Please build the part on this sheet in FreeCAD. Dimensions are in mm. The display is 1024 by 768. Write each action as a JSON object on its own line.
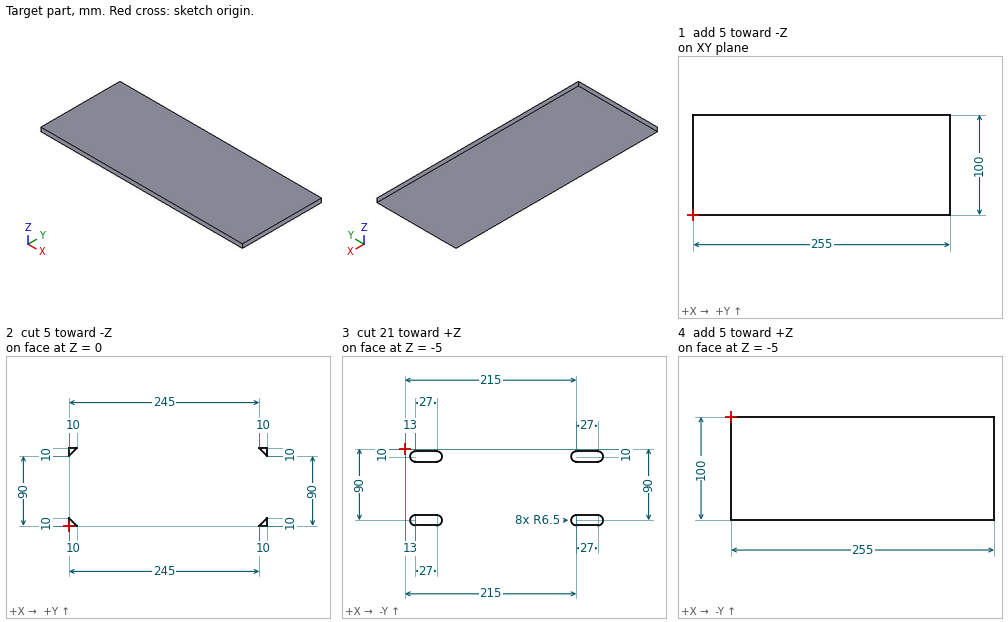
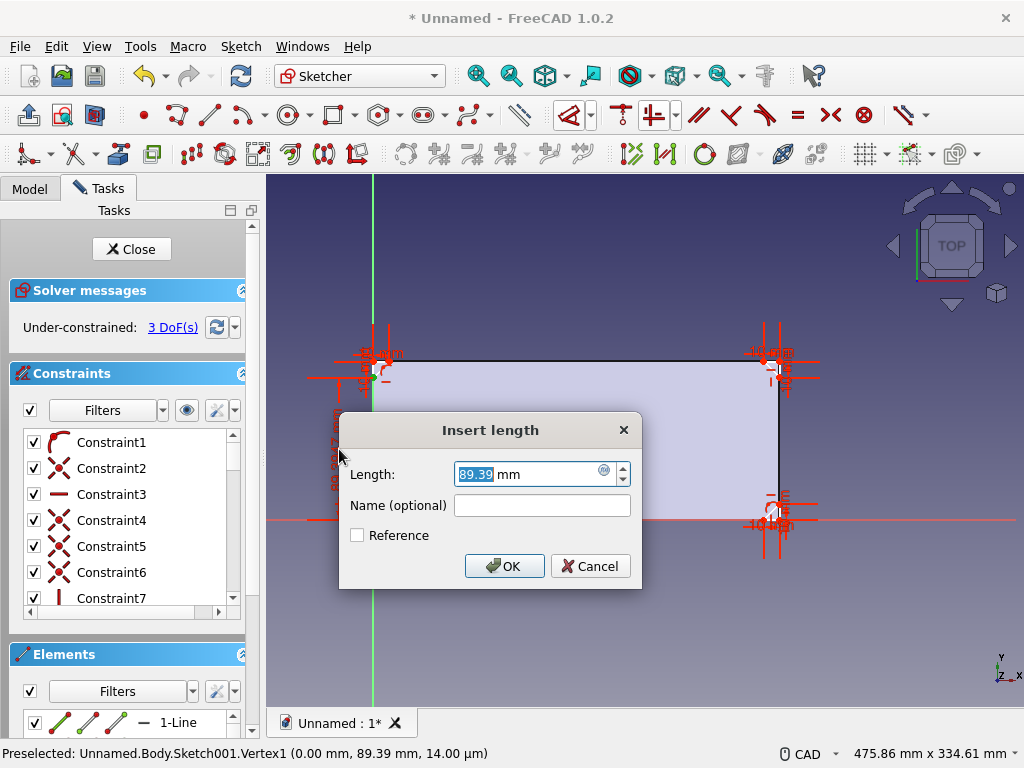
{"action": "type", "text": "90"}
{"action": "key", "text": "Return"}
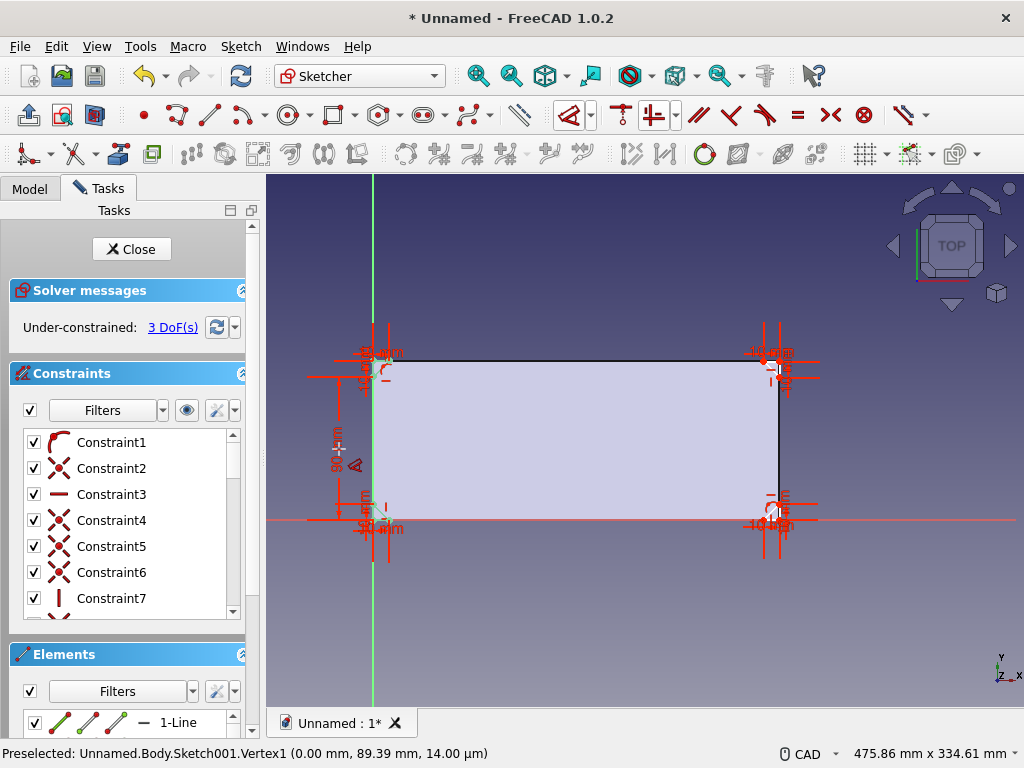
{"action": "left_click", "coordinate": [780, 378]}
{"action": "left_click", "coordinate": [814, 449]}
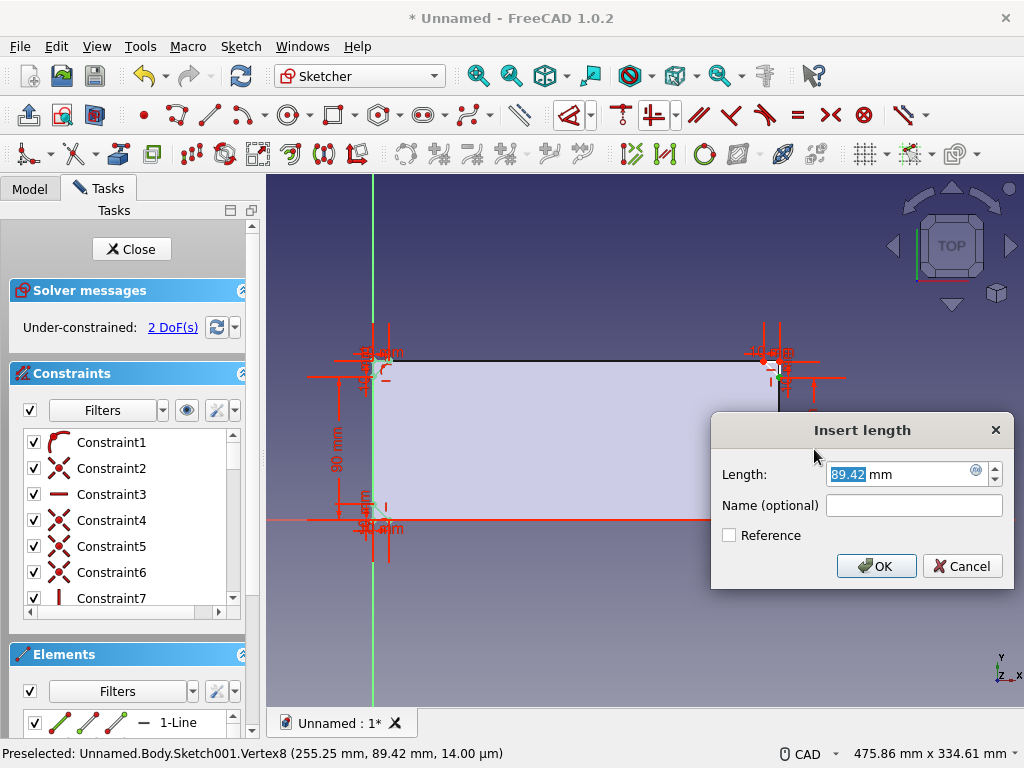
{"action": "type", "text": "90"}
{"action": "key", "text": "Return"}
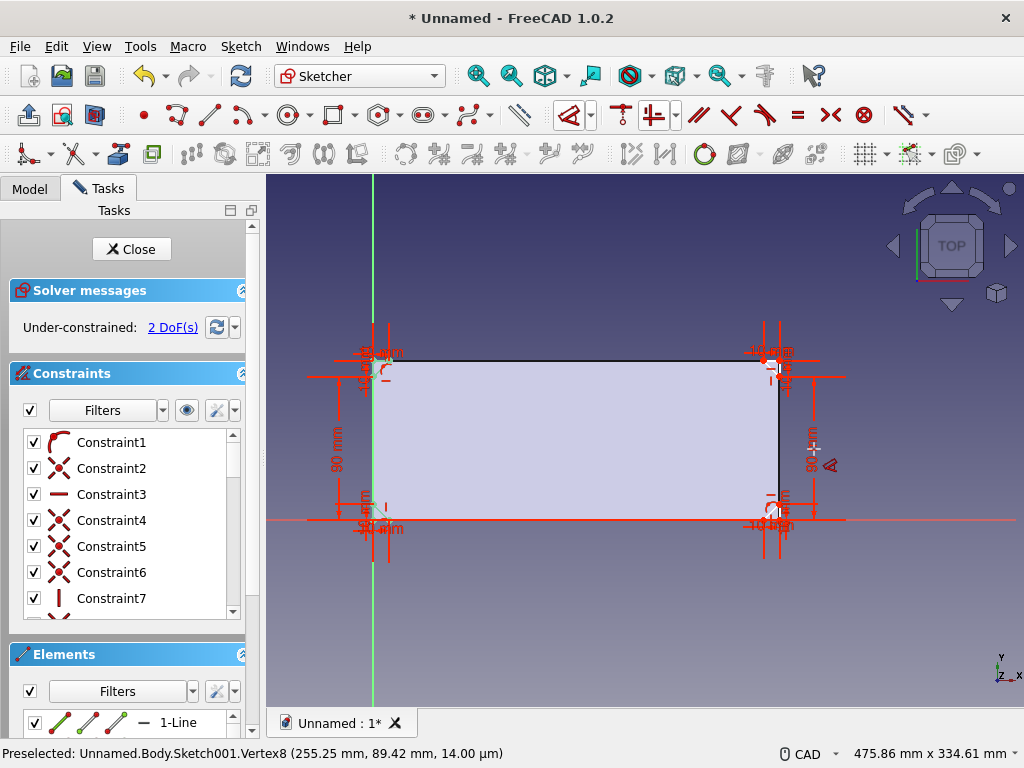
{"action": "left_click", "coordinate": [764, 361]}
{"action": "left_click", "coordinate": [569, 554]}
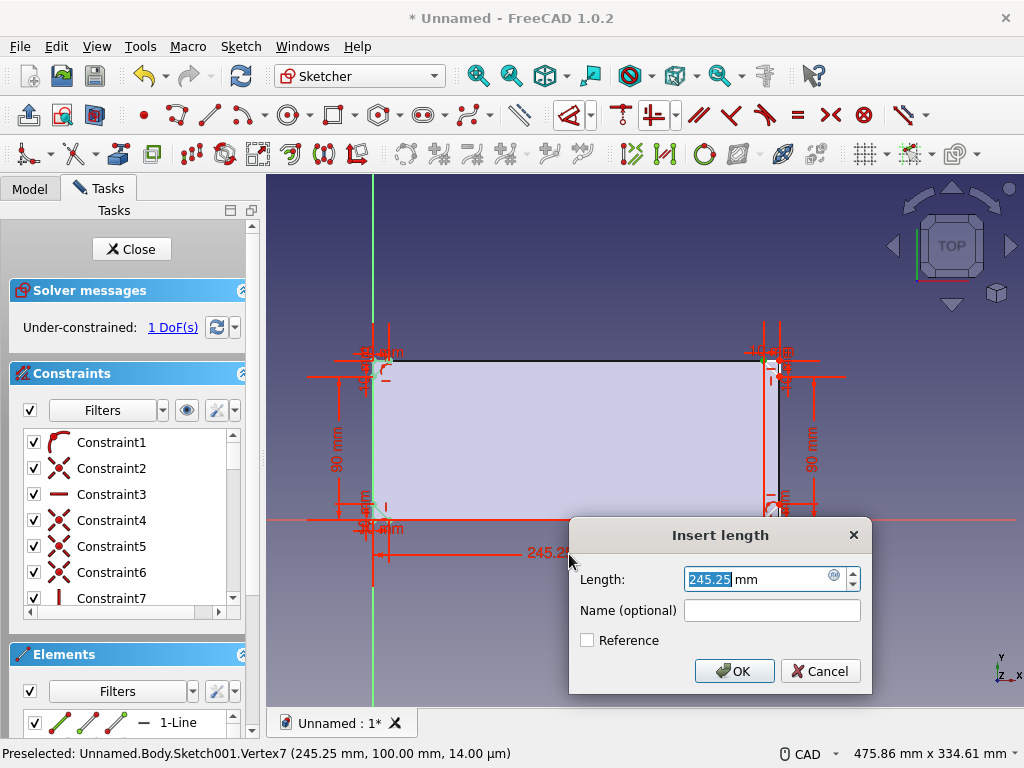
{"action": "type", "text": "245"}
{"action": "key", "text": "Return"}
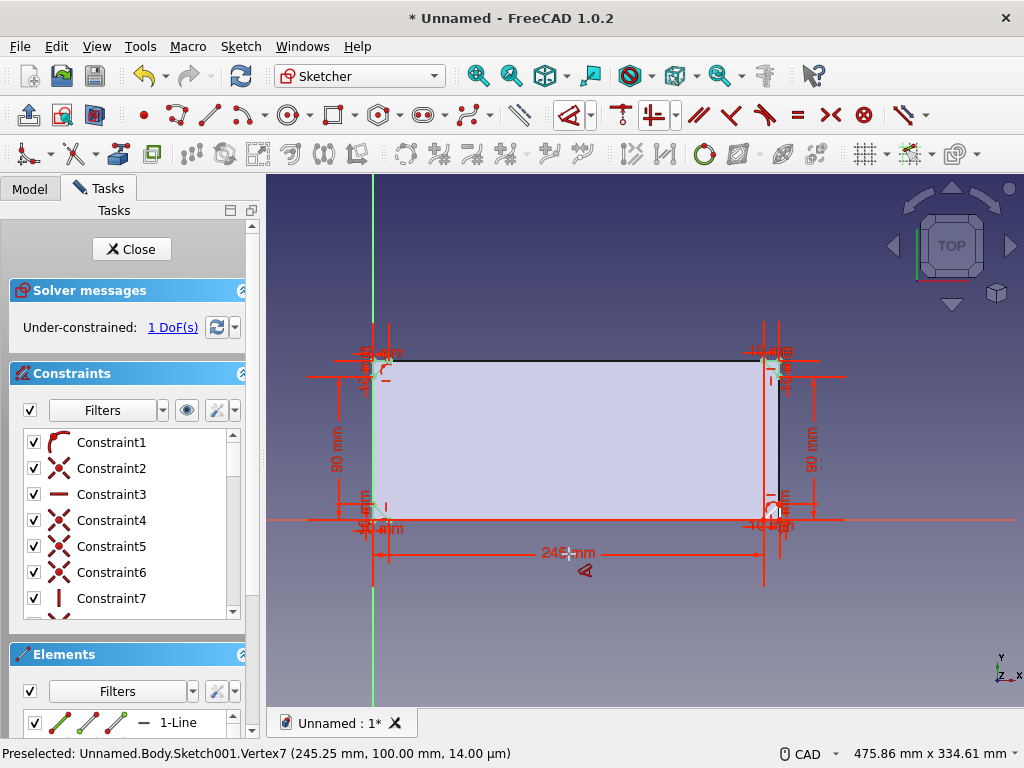
{"action": "left_click", "coordinate": [764, 520]}
{"action": "left_click", "coordinate": [479, 554]}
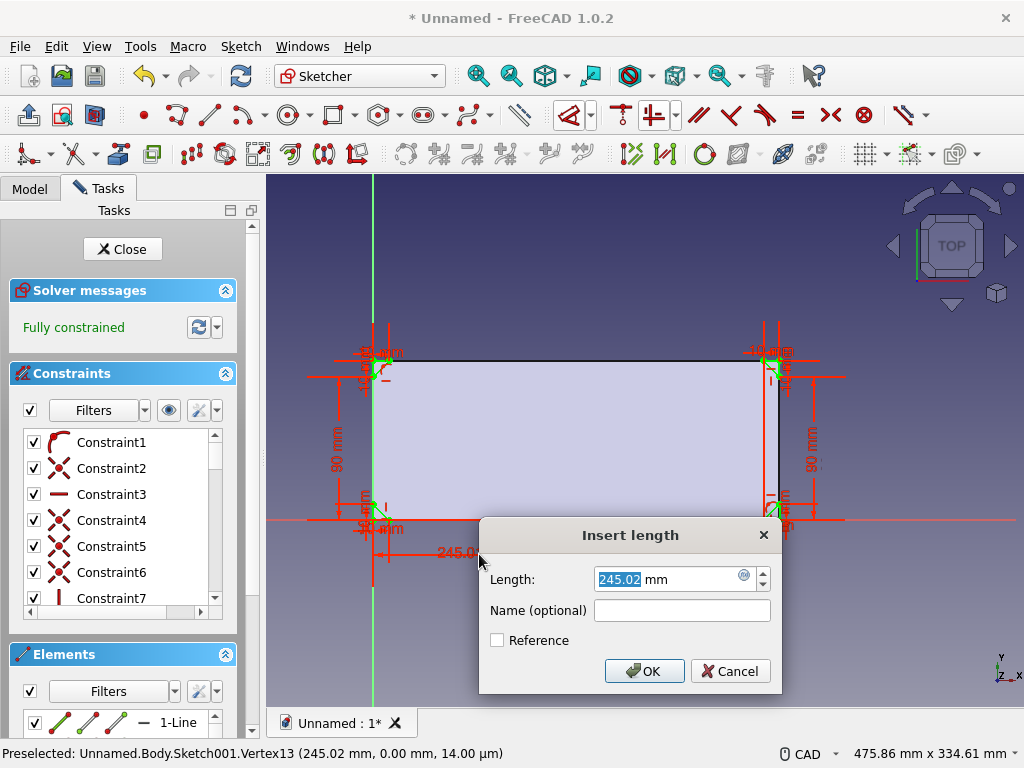
{"action": "type", "text": "245"}
{"action": "key", "text": "Return"}
{"action": "key", "text": "Escape"}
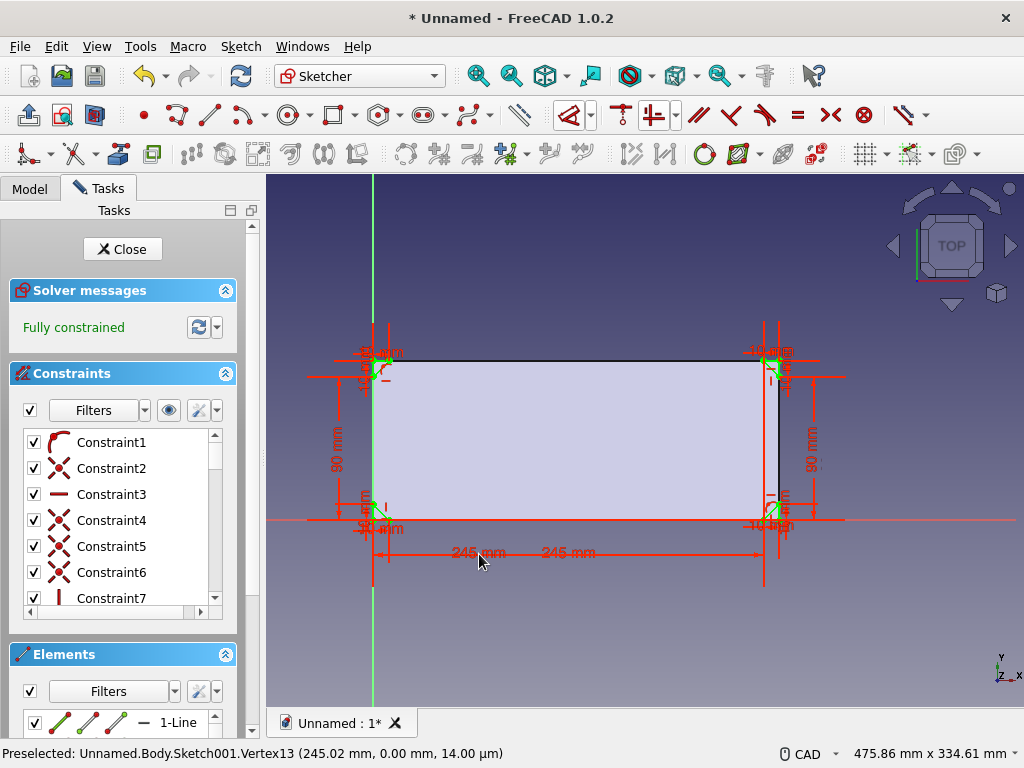
{"action": "left_click", "coordinate": [123, 249]}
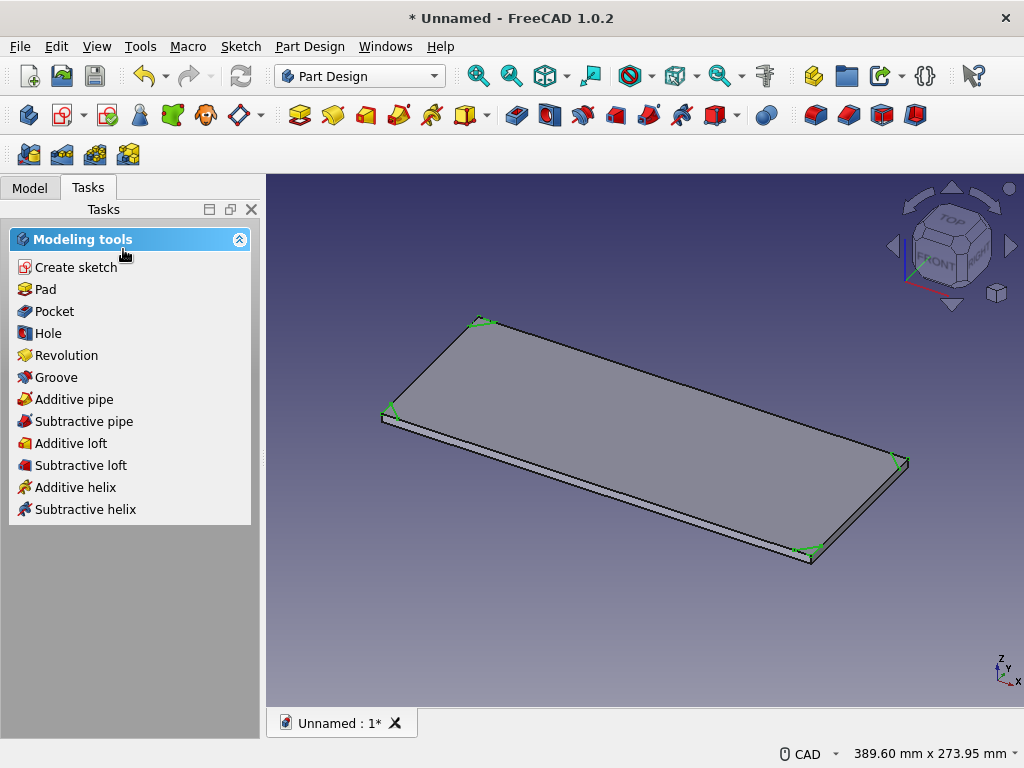
{"action": "left_click", "coordinate": [517, 116]}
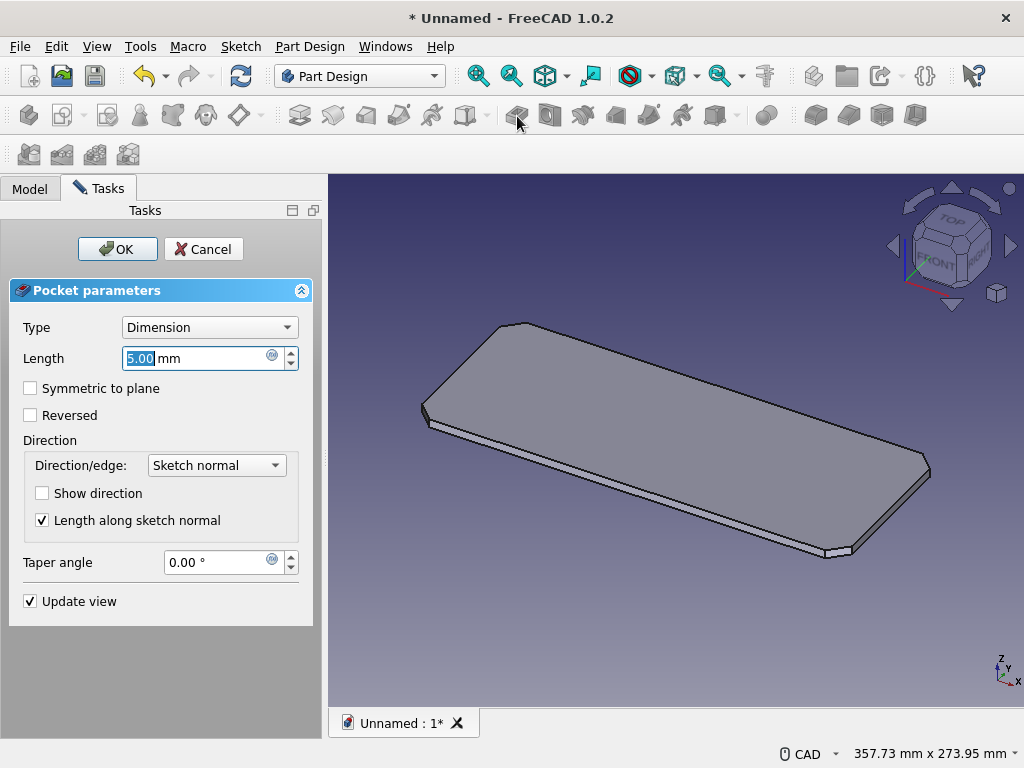
{"action": "type", "text": "5"}
{"action": "key", "text": "Tab"}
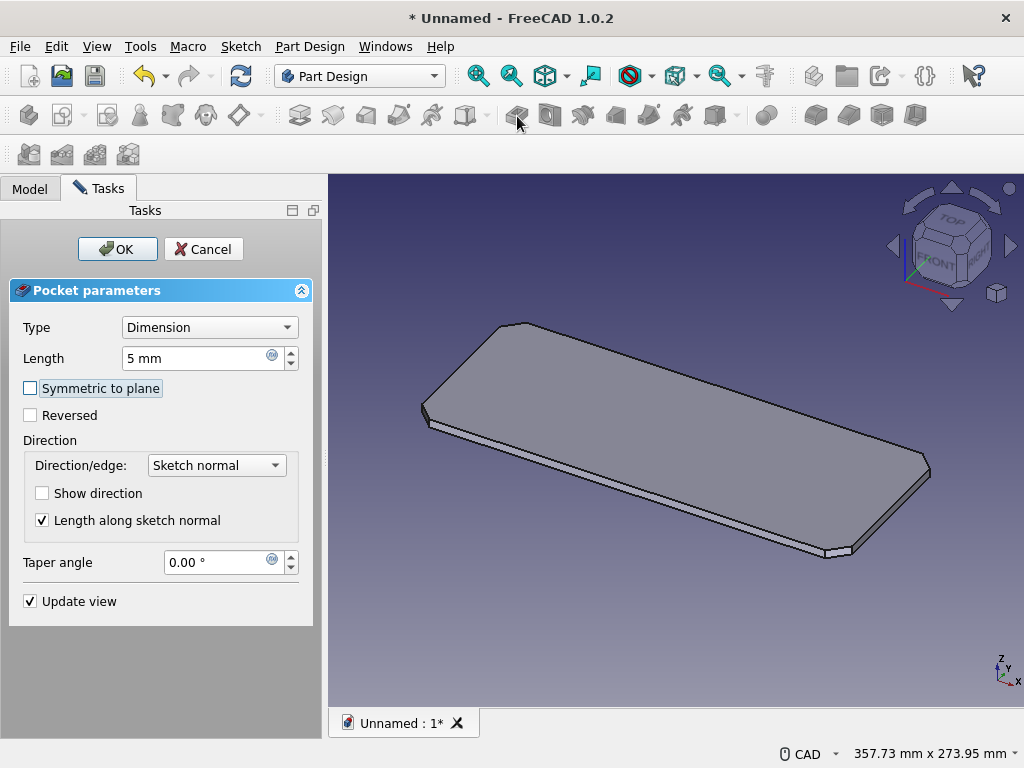
{"action": "left_click", "coordinate": [118, 249]}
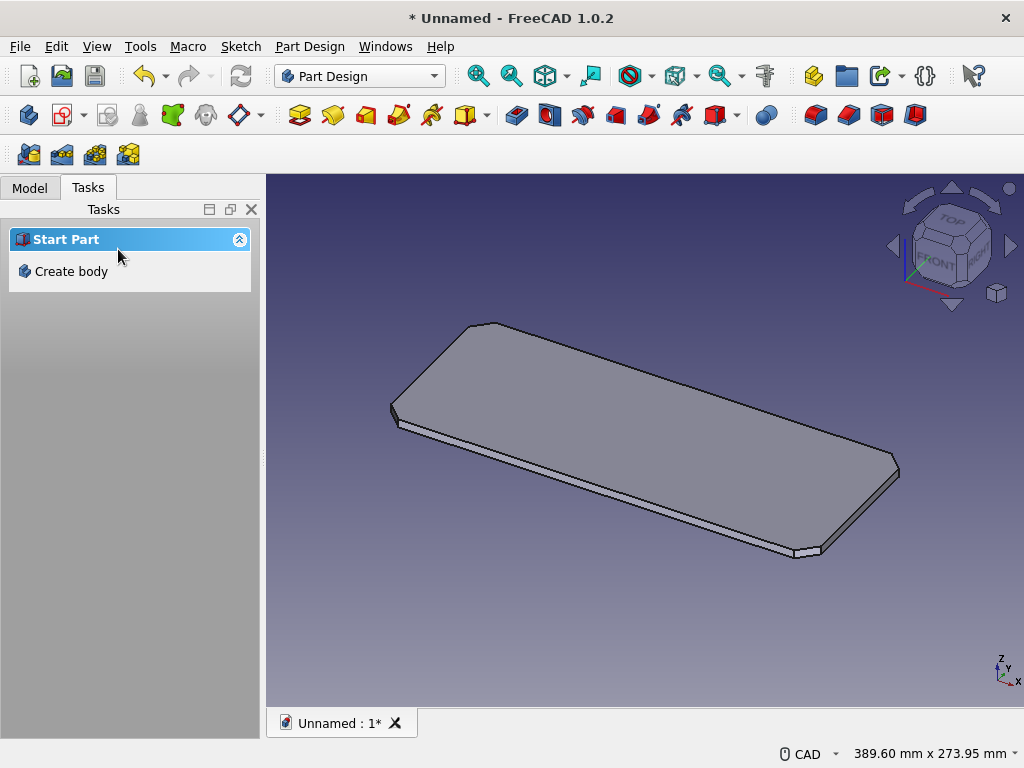
{"action": "key", "text": "5"}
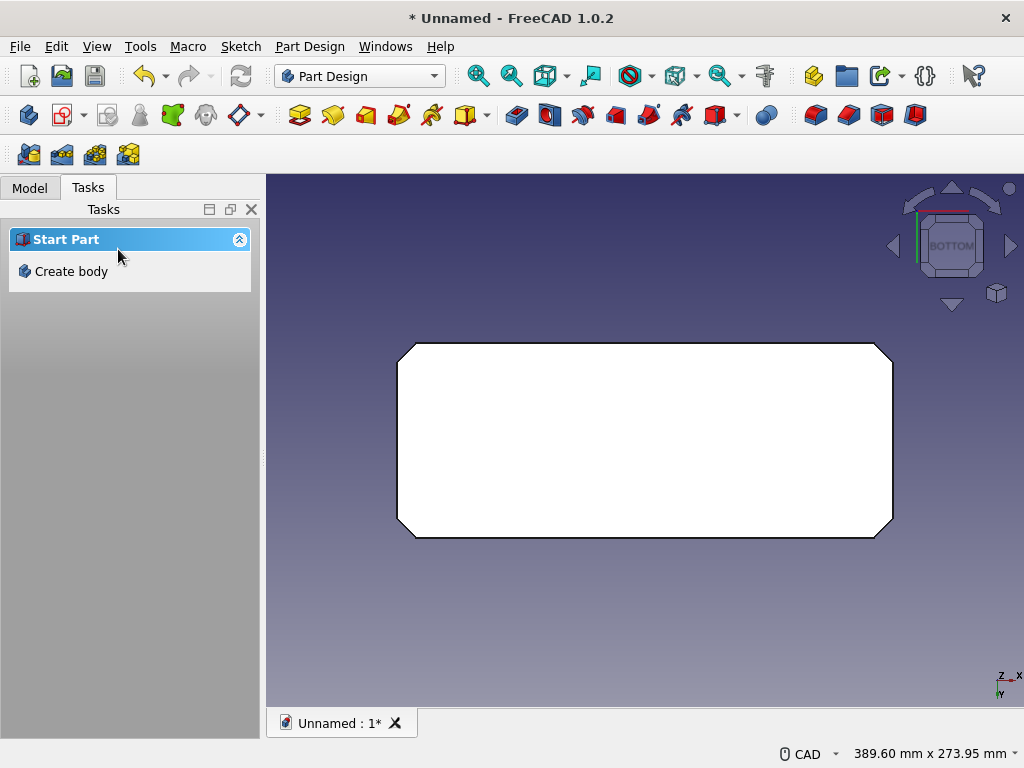
{"action": "left_click", "coordinate": [787, 439]}